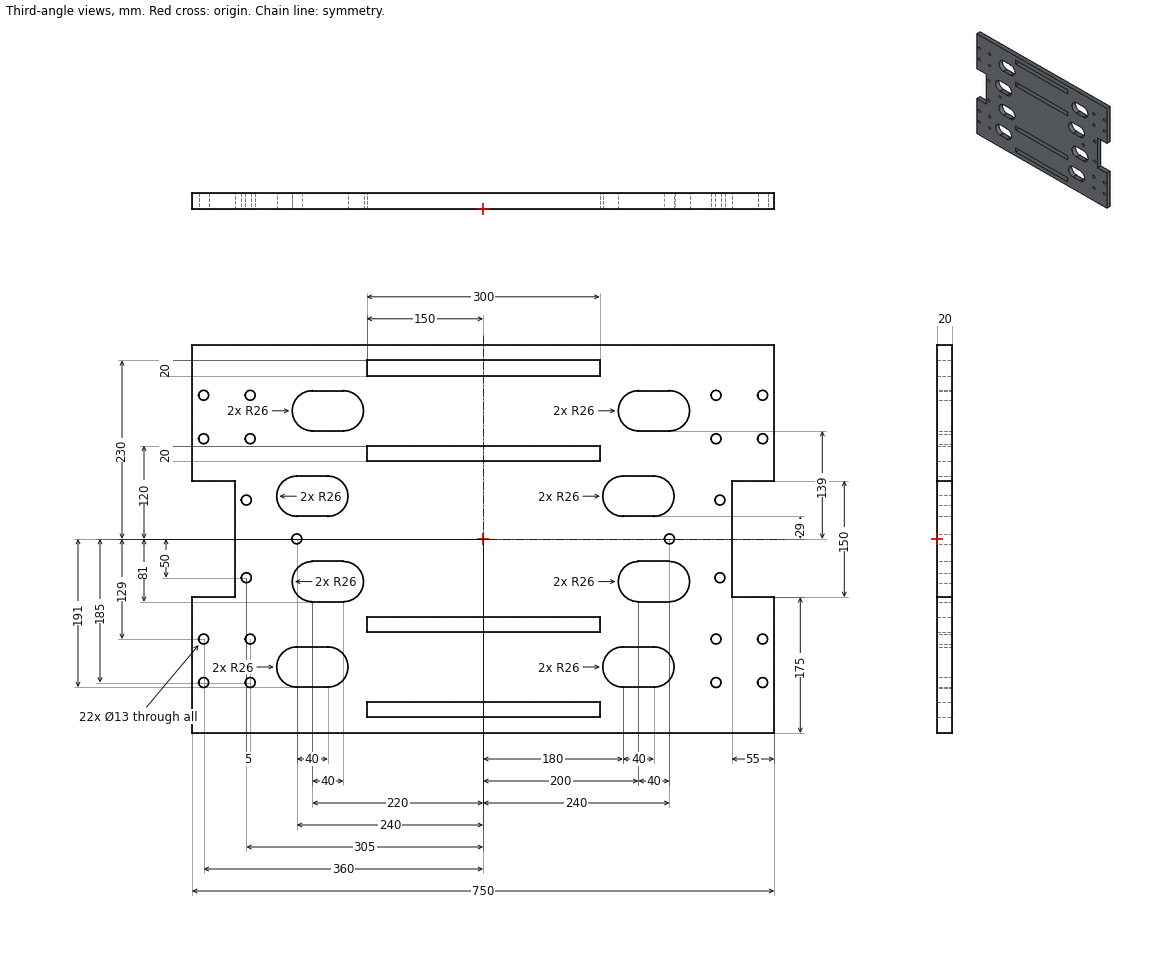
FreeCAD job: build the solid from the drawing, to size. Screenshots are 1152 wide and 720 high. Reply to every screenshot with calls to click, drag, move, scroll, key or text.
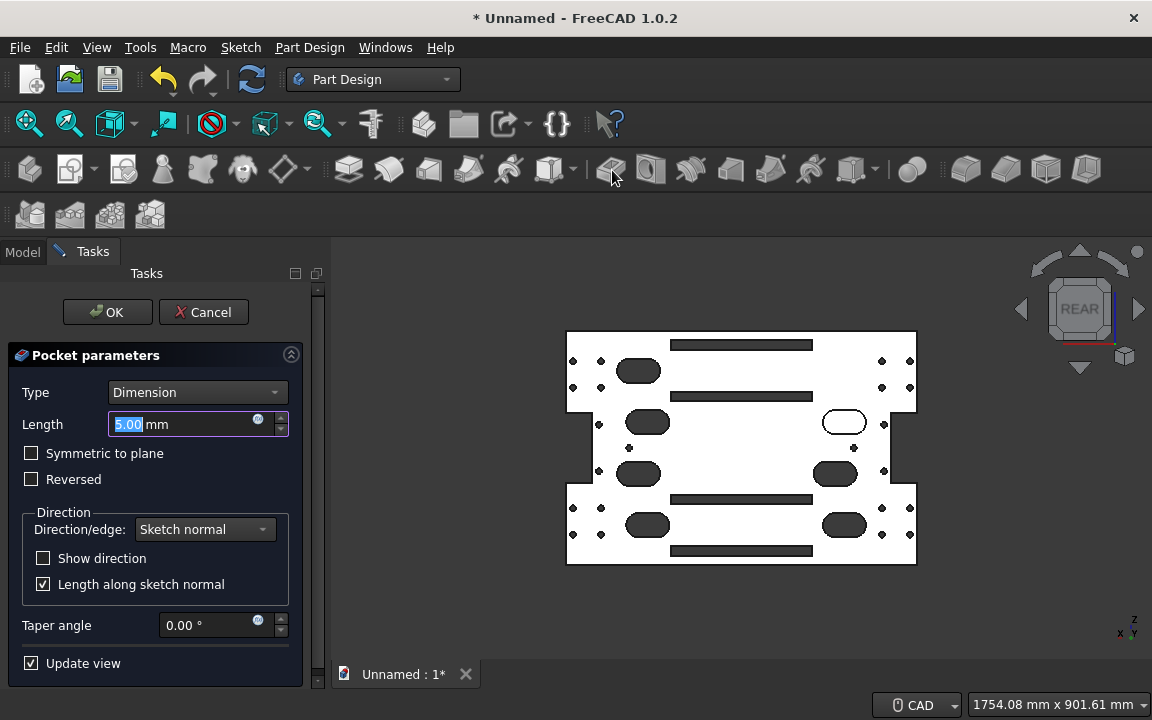
click(198, 392)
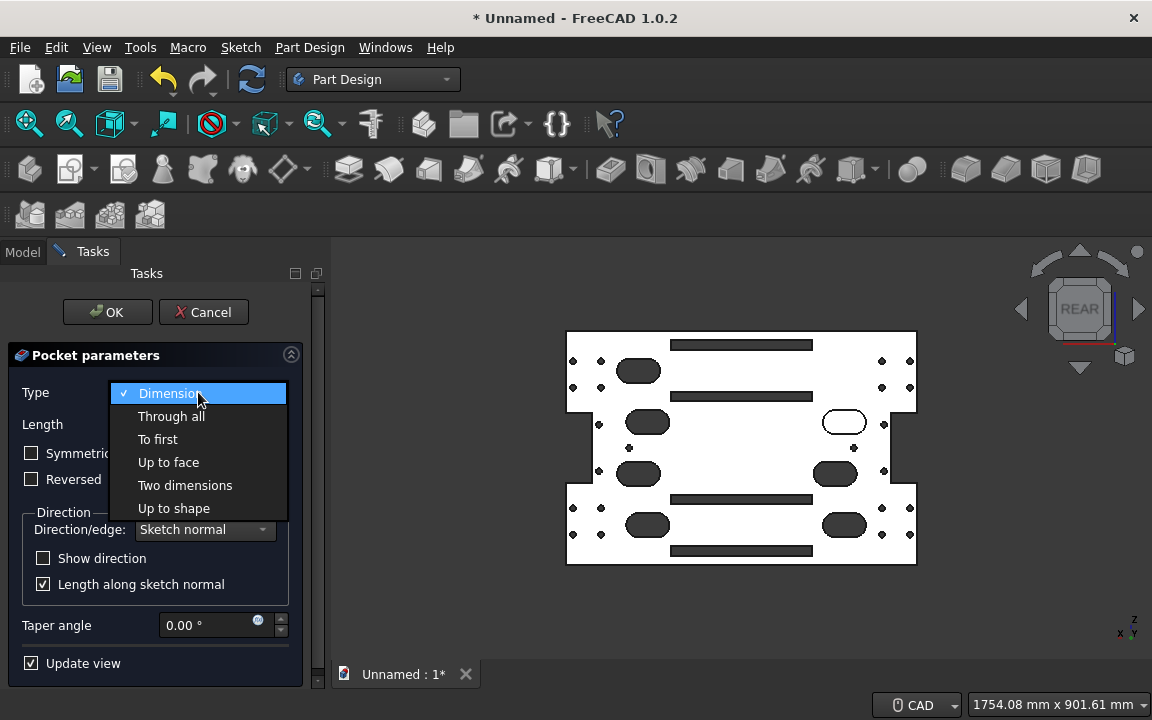
click(198, 440)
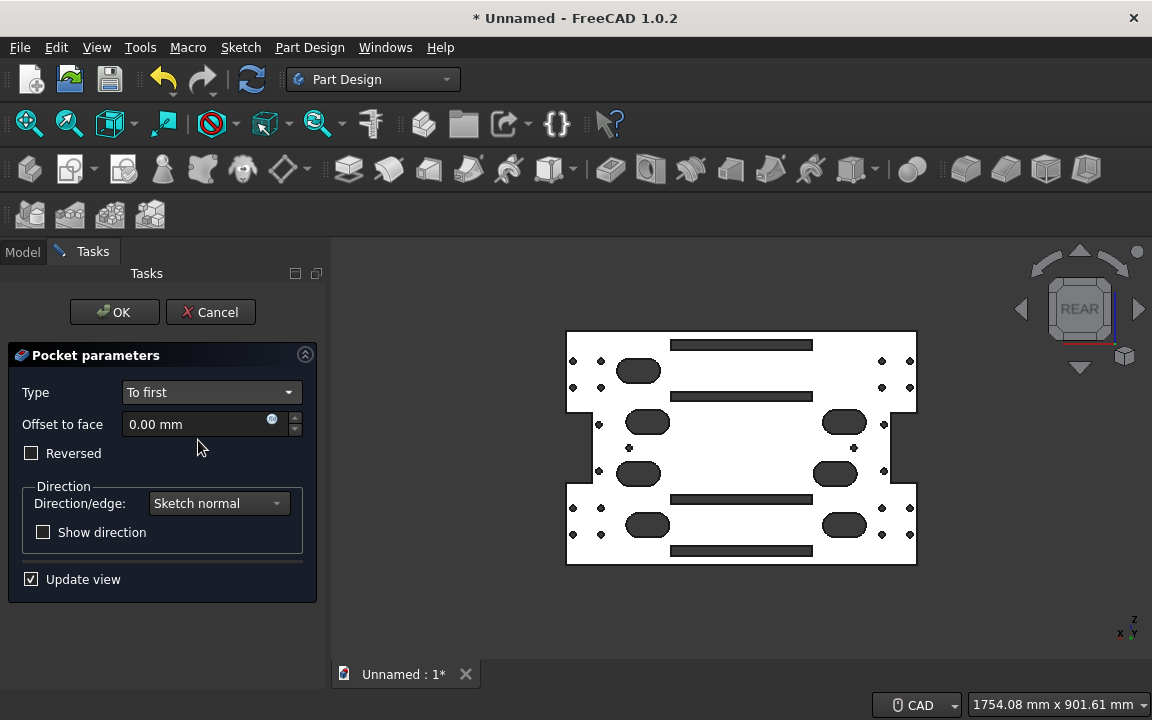
click(115, 312)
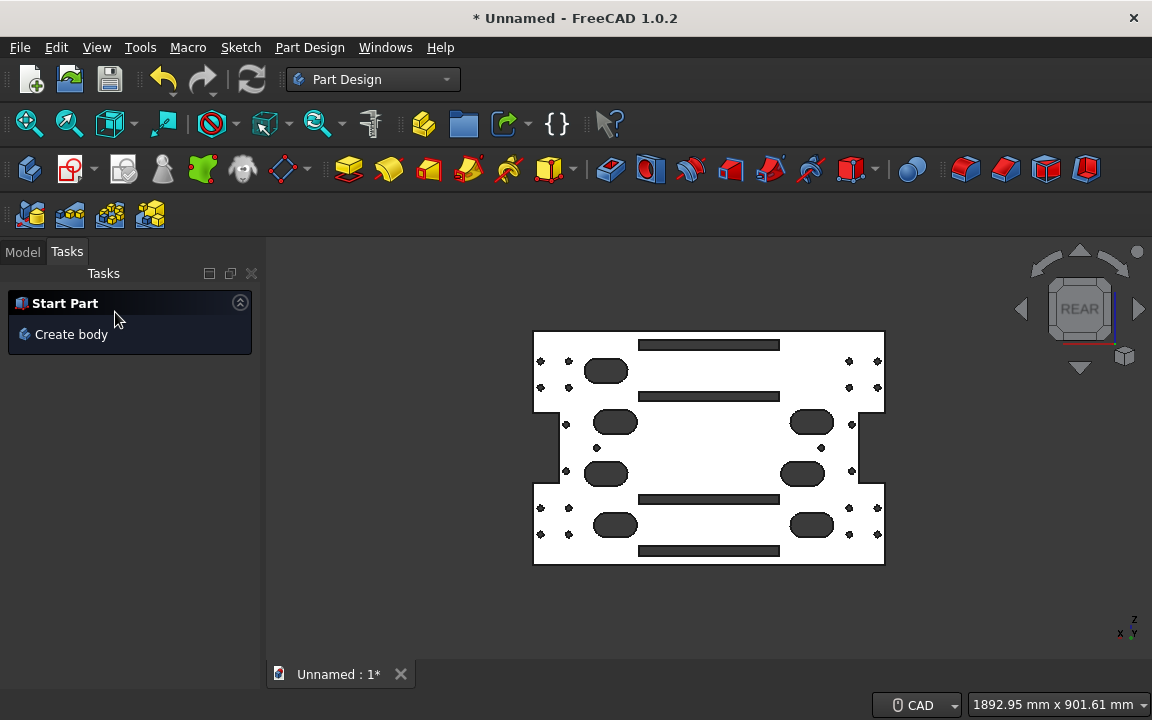
click(709, 447)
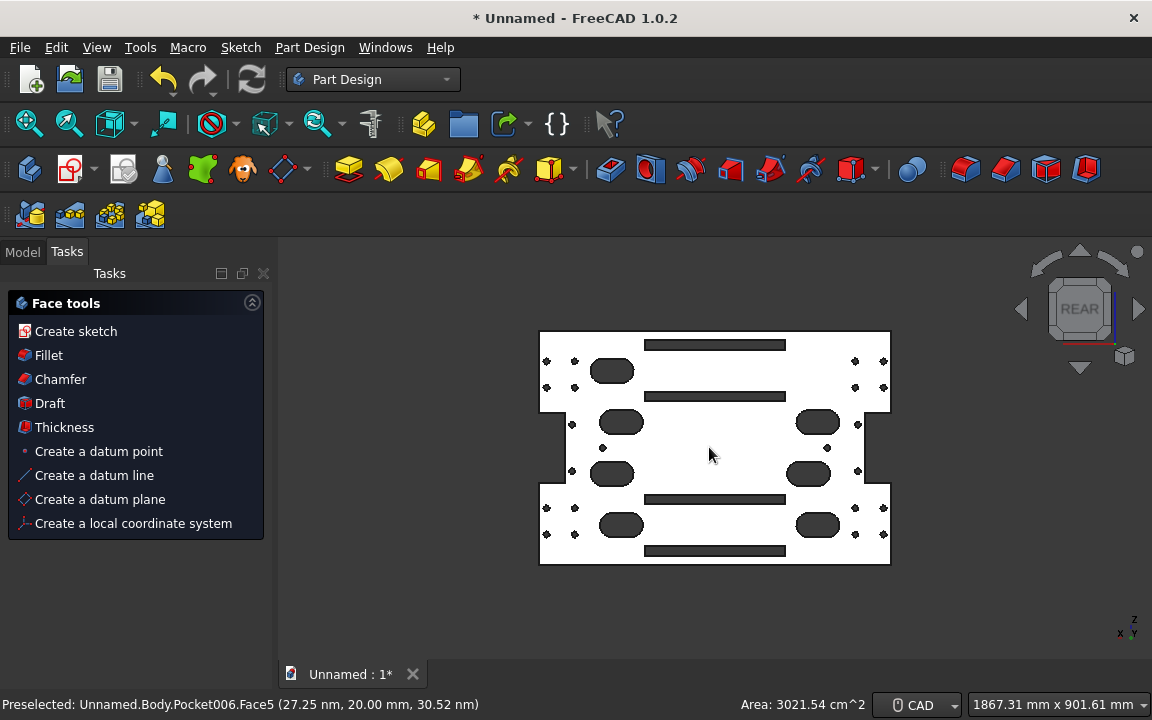
click(70, 170)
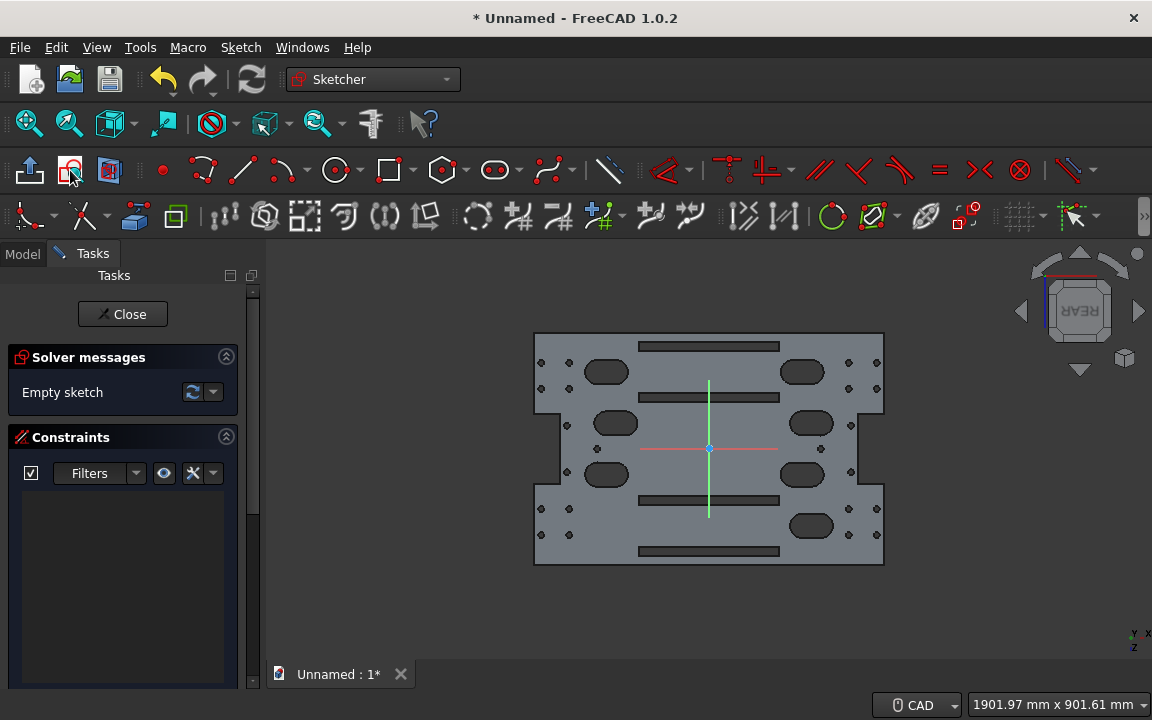
scroll(613, 534, up, 12)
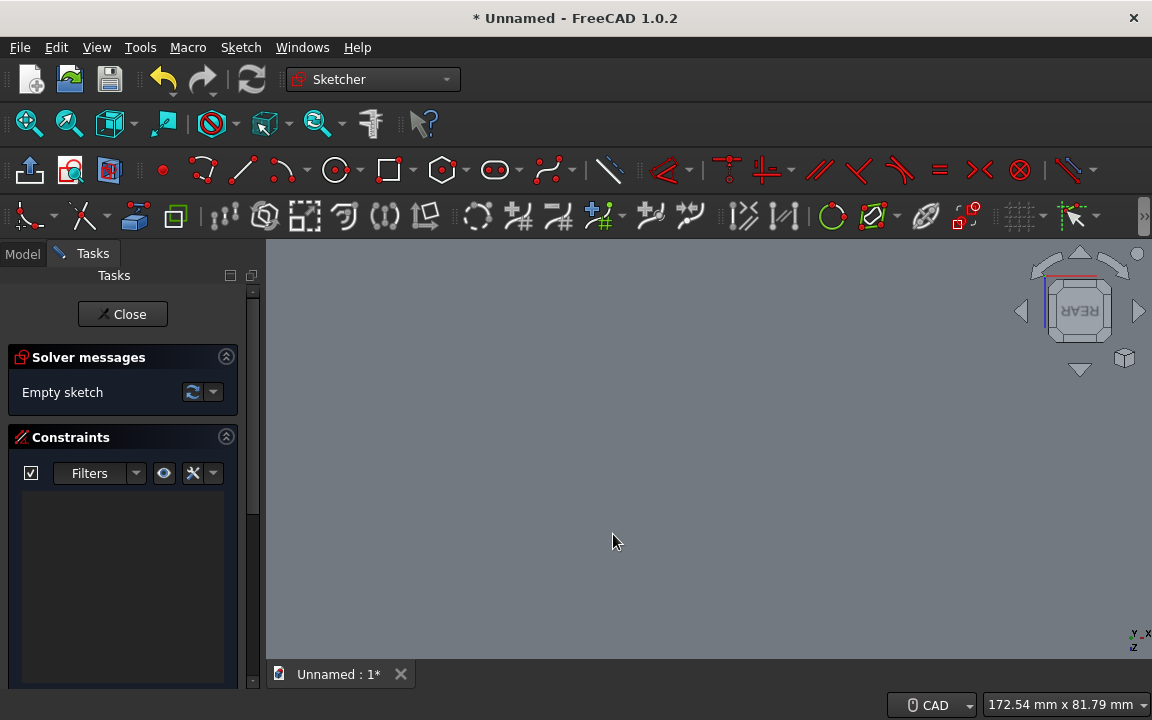
click(496, 170)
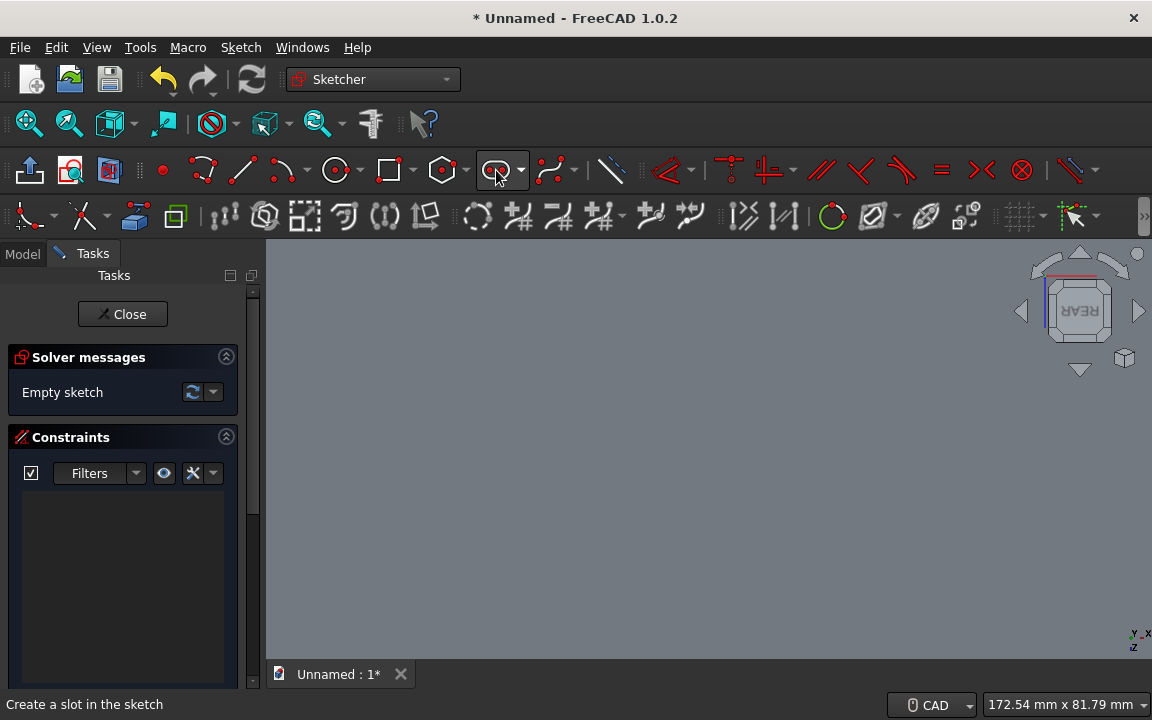
click(538, 437)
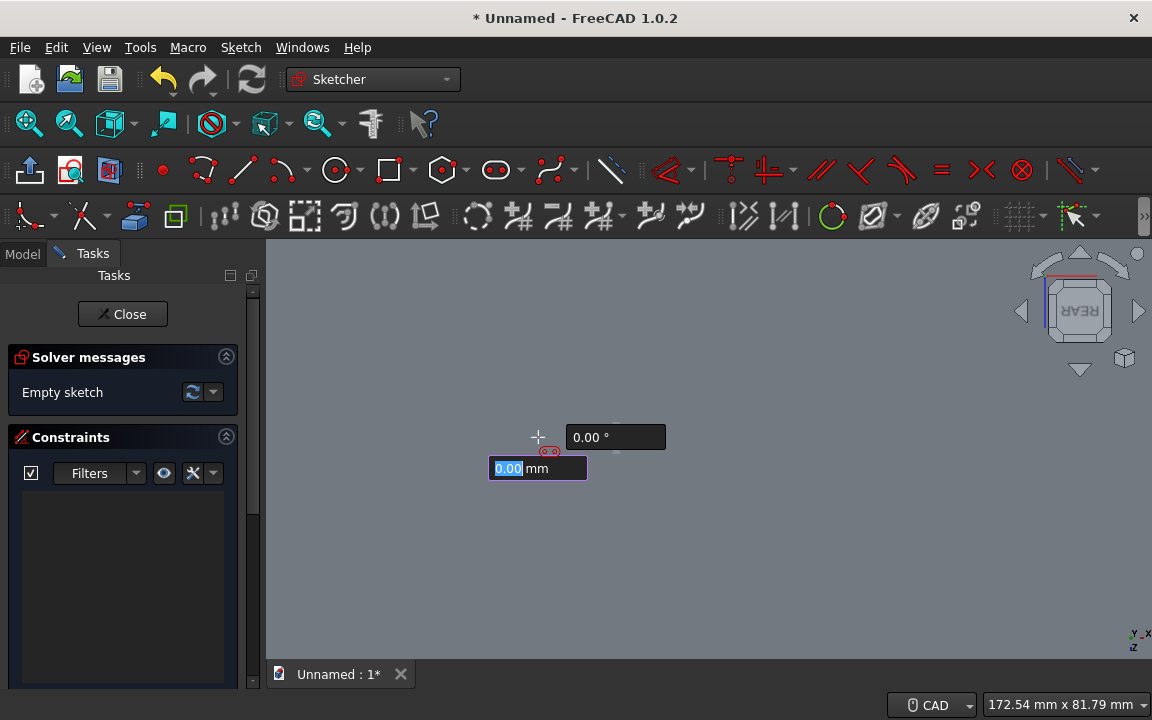
click(743, 437)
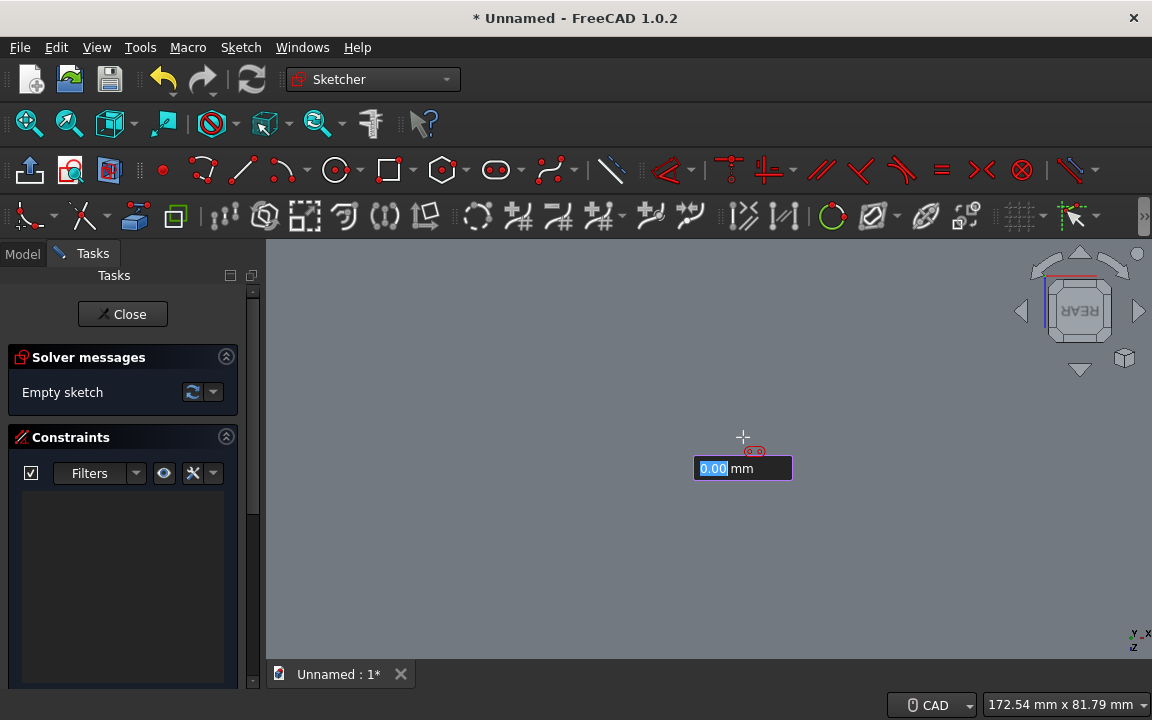
click(640, 304)
key(Escape)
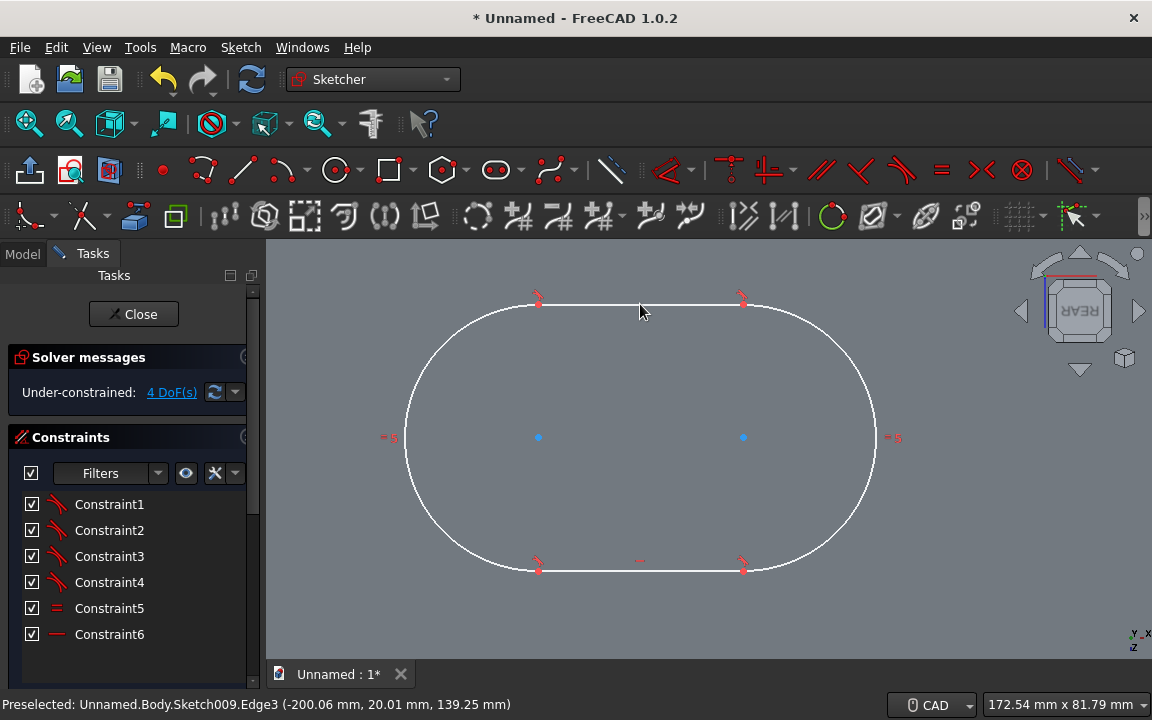
click(666, 170)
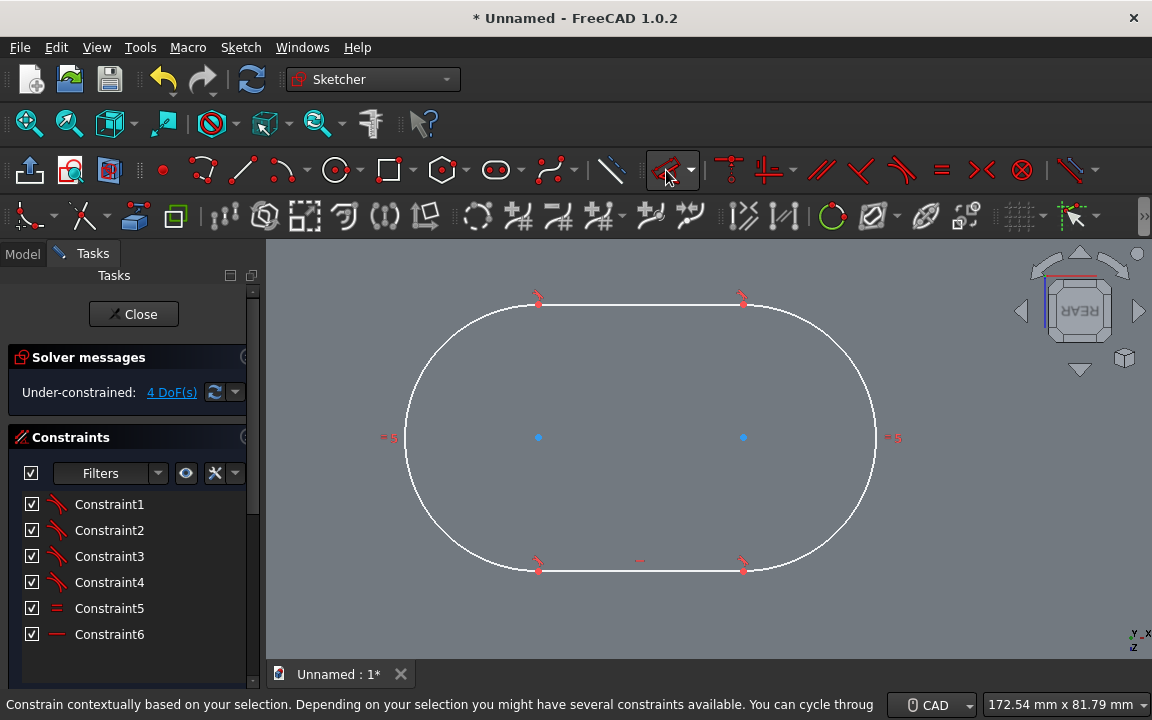
click(430, 360)
click(404, 341)